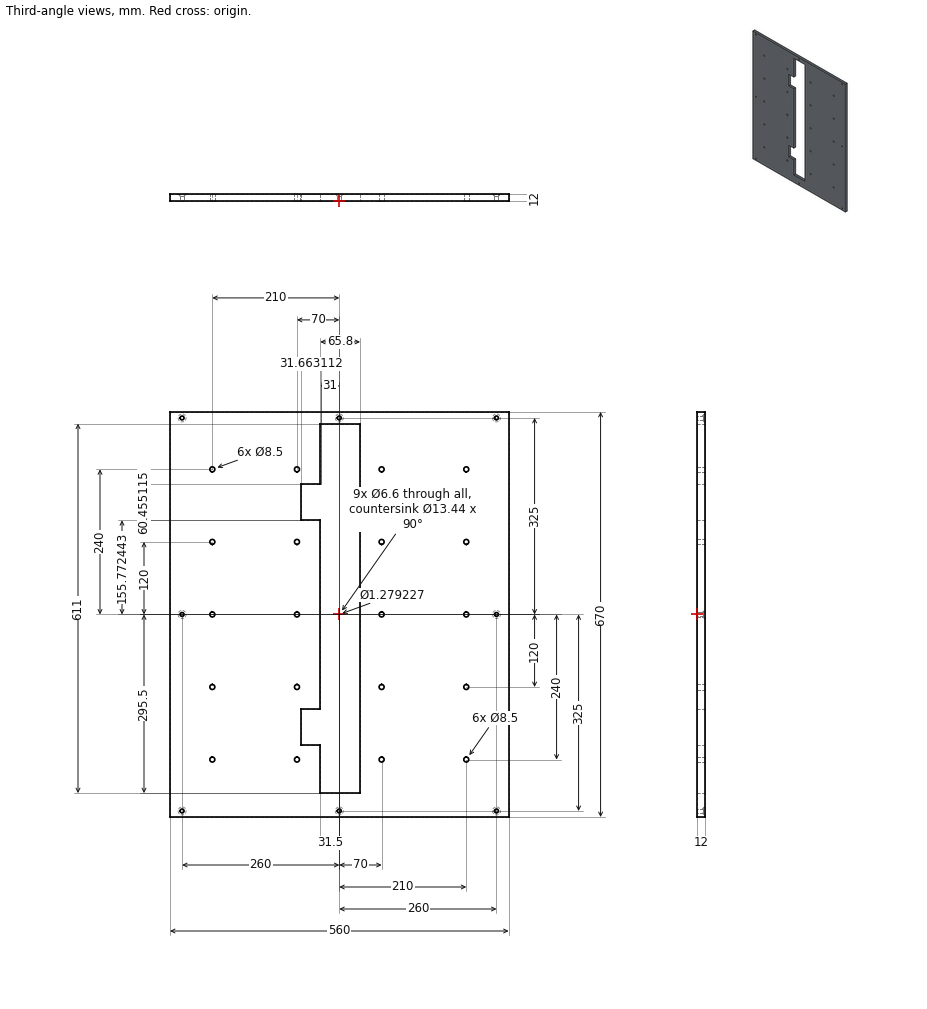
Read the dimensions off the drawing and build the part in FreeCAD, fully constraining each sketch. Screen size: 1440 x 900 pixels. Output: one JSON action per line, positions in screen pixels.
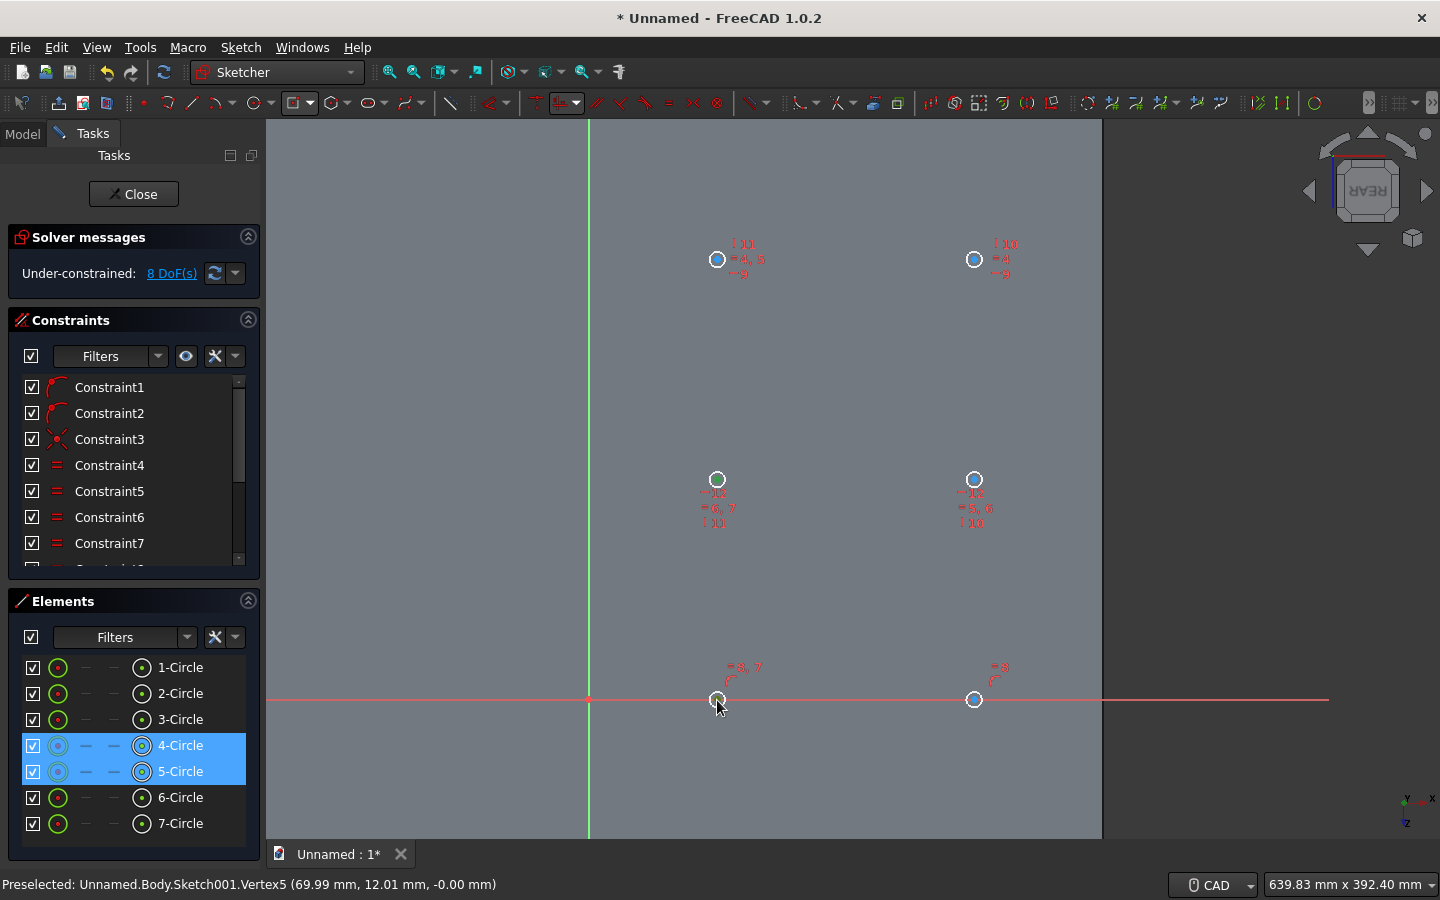
{"action": "left_click", "coordinate": [578, 104]}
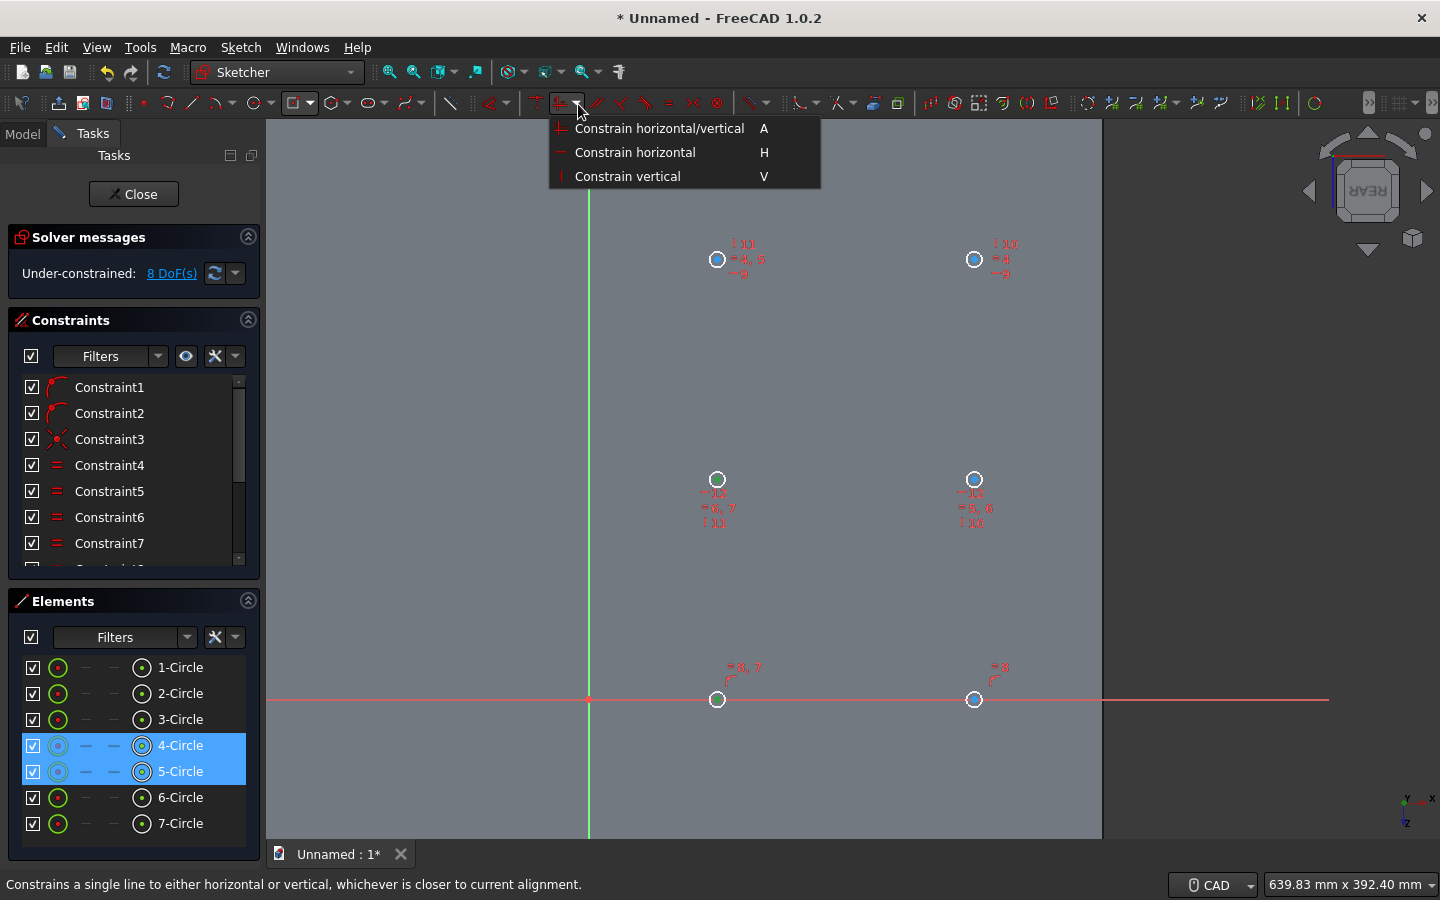
{"action": "left_click", "coordinate": [685, 176]}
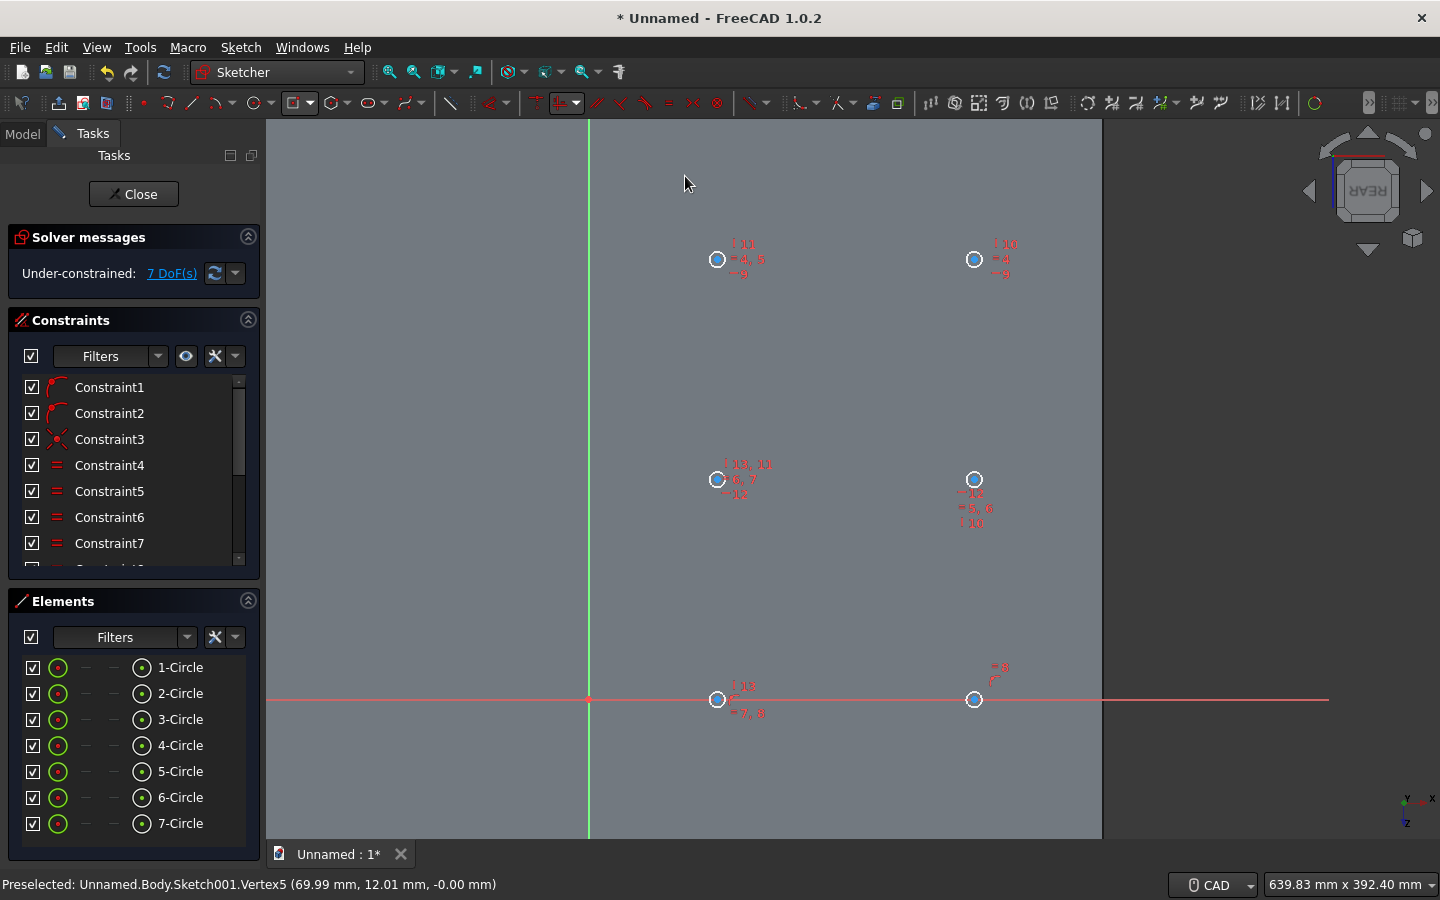
{"action": "left_click", "coordinate": [974, 480]}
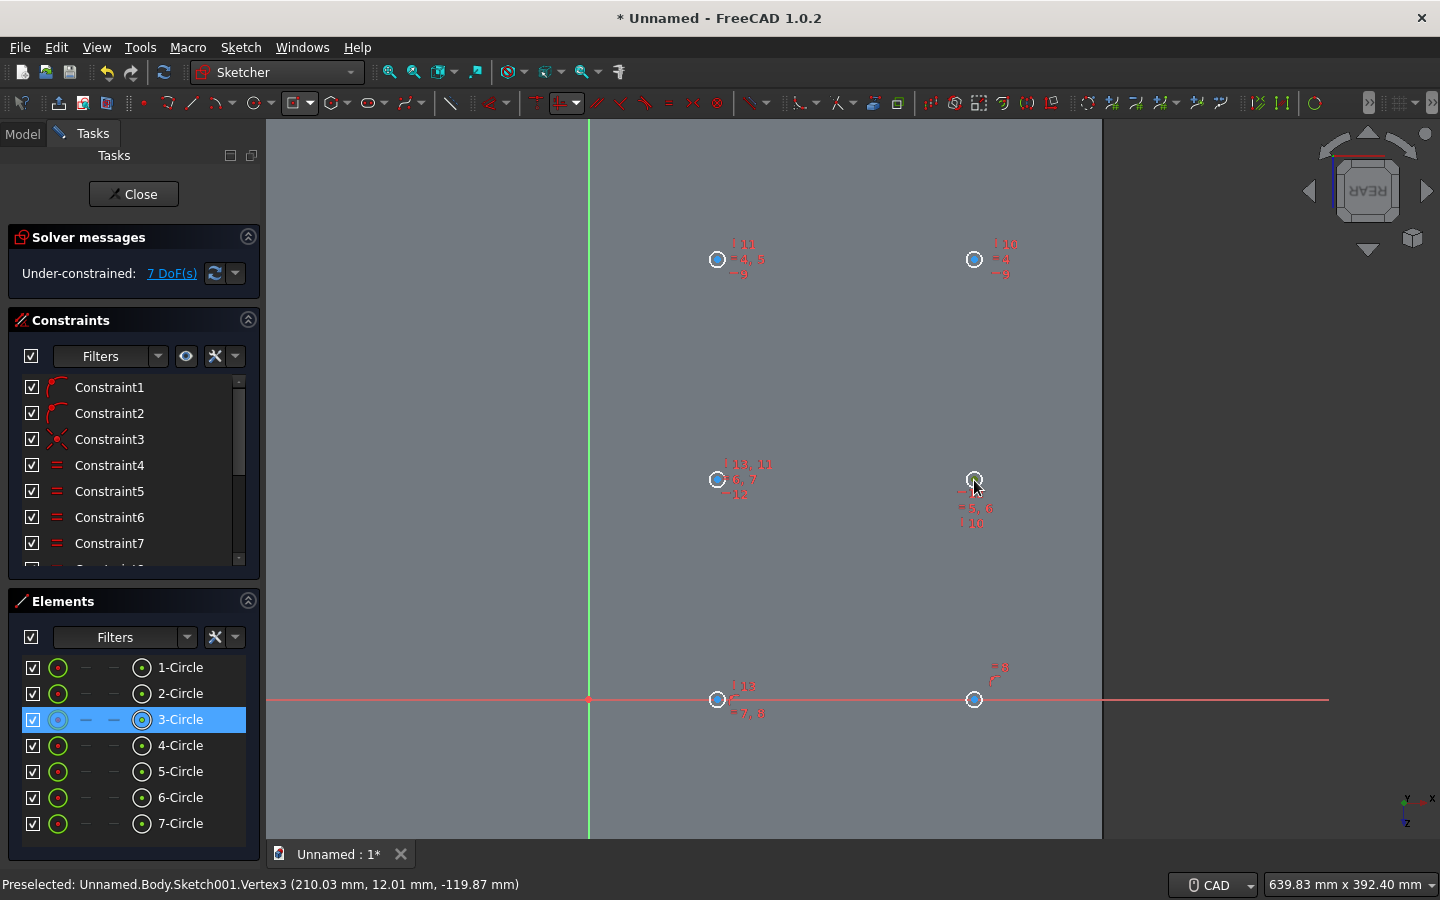
{"action": "left_click", "coordinate": [974, 700]}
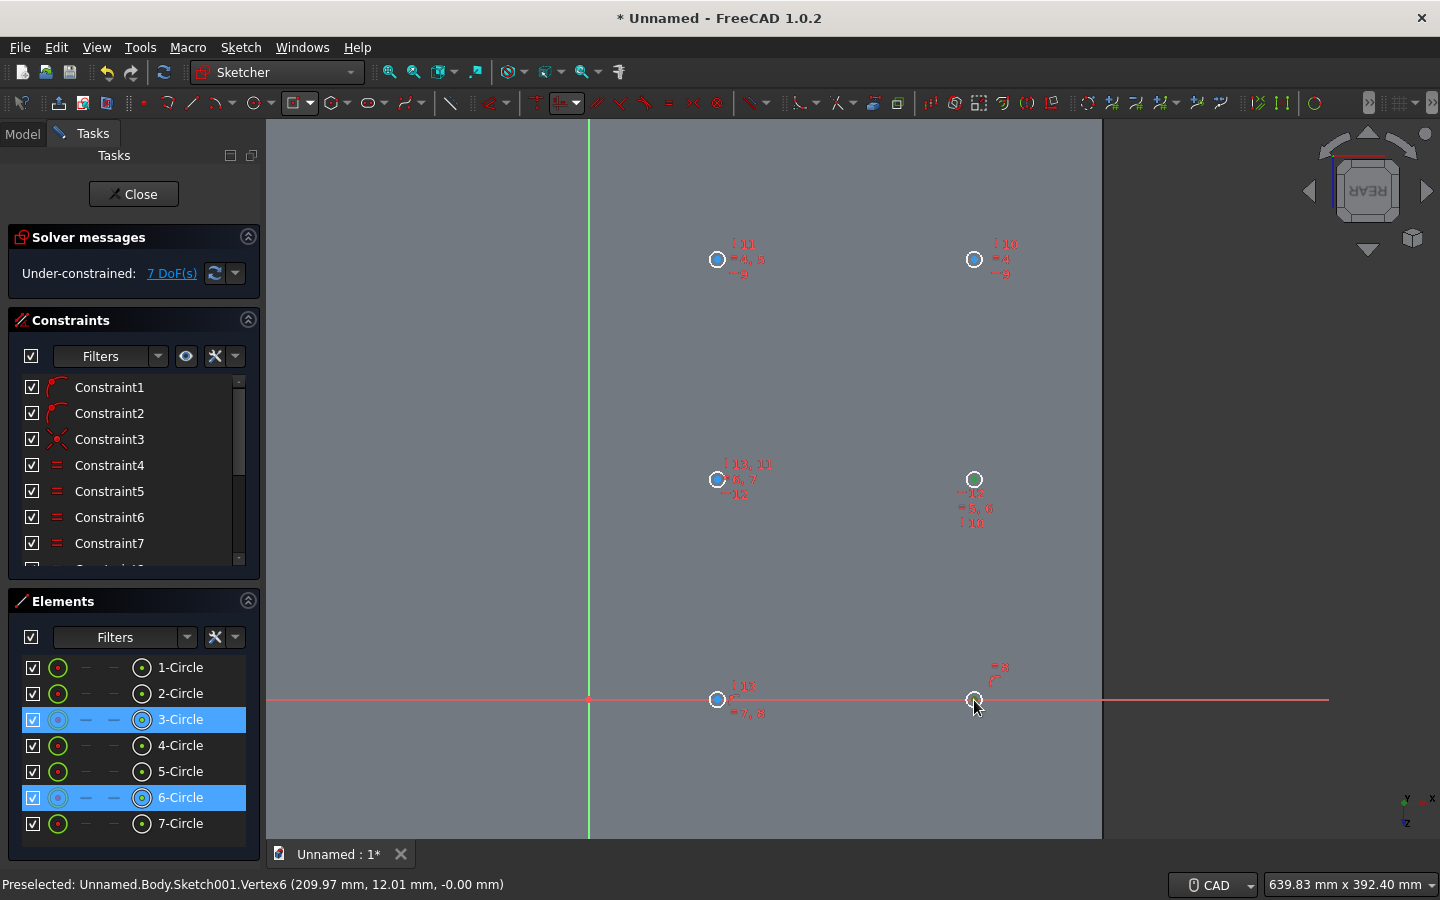
{"action": "left_click", "coordinate": [578, 104]}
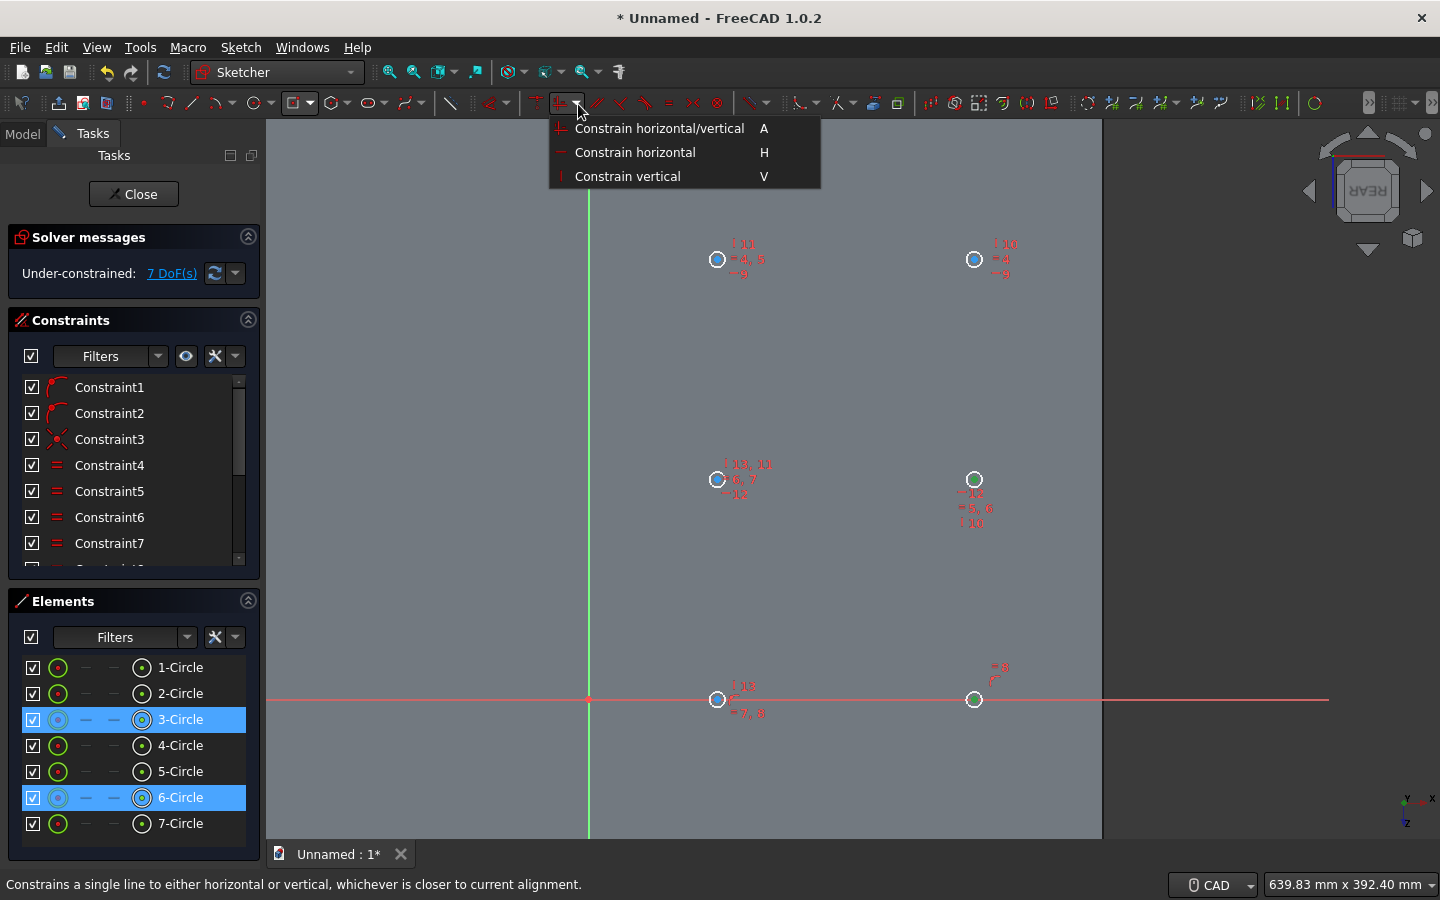
{"action": "left_click", "coordinate": [685, 176]}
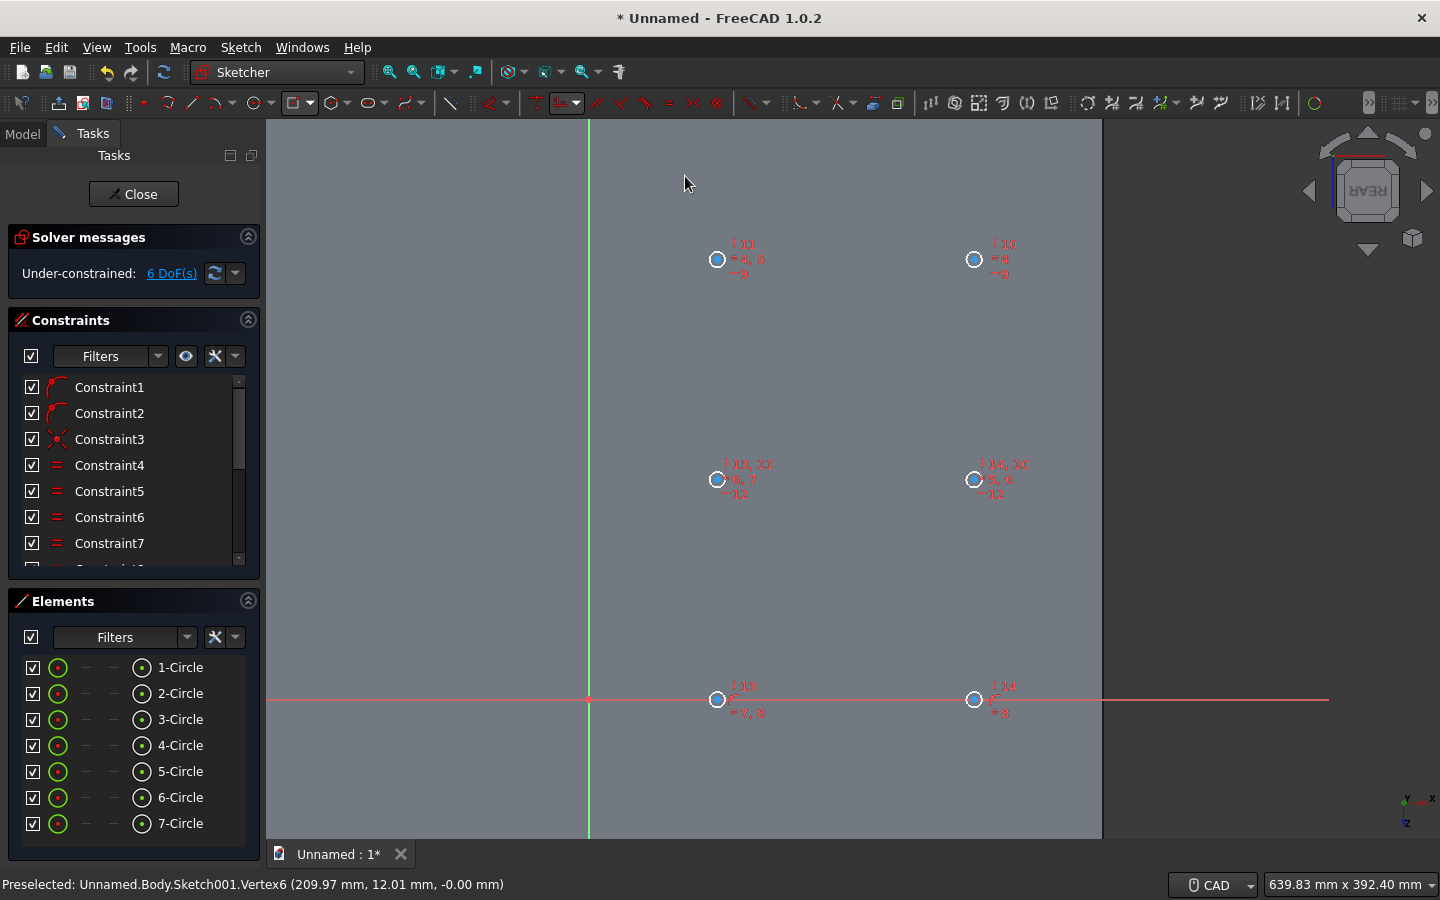
{"action": "left_click", "coordinate": [490, 104]}